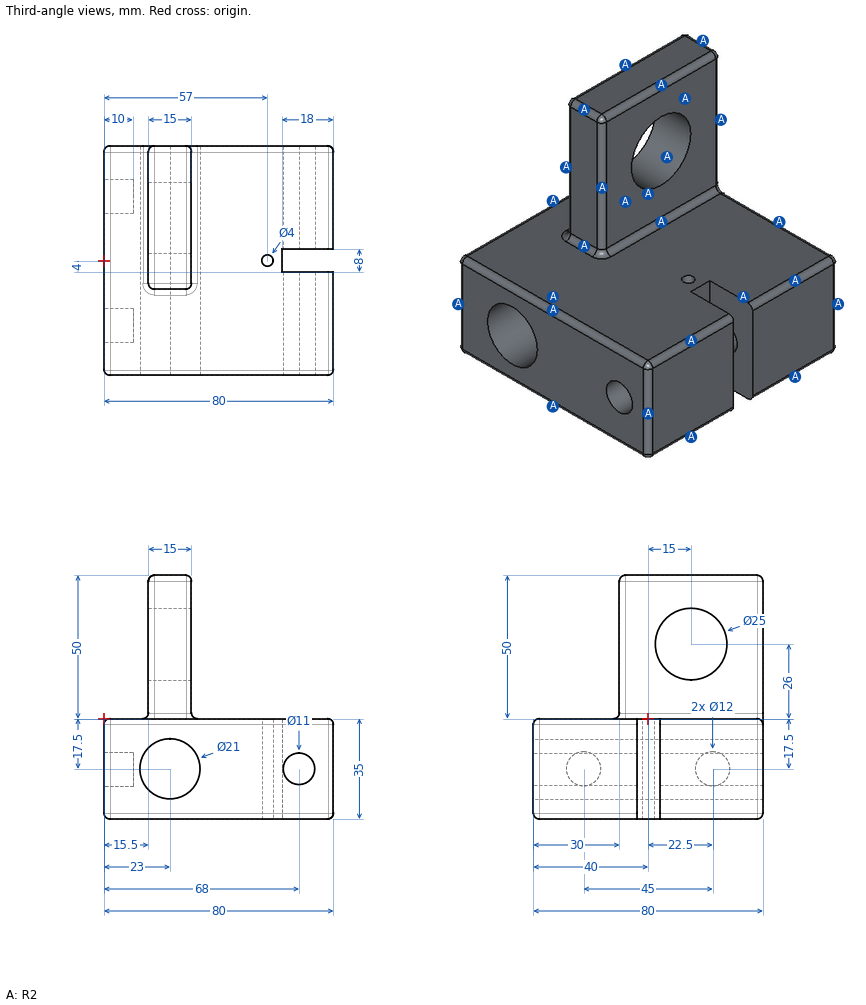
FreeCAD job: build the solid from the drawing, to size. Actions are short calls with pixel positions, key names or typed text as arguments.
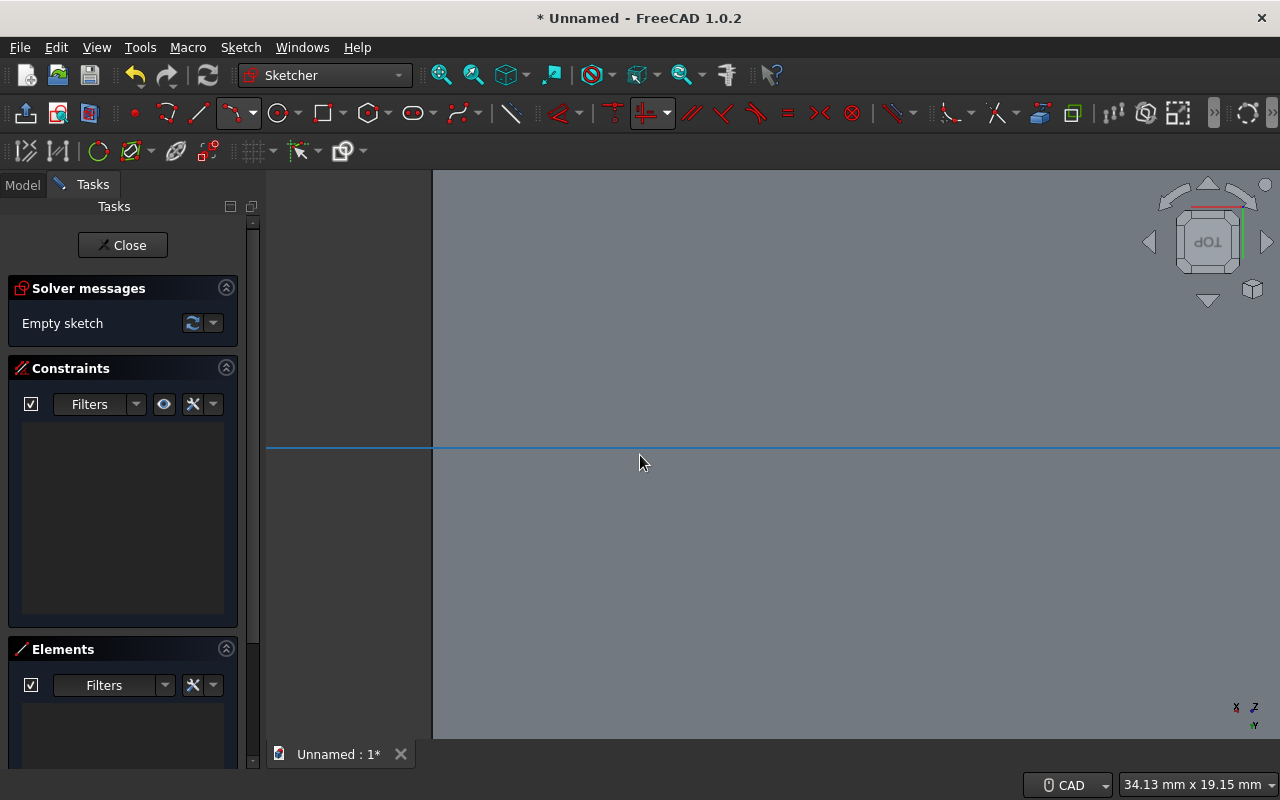
click(324, 114)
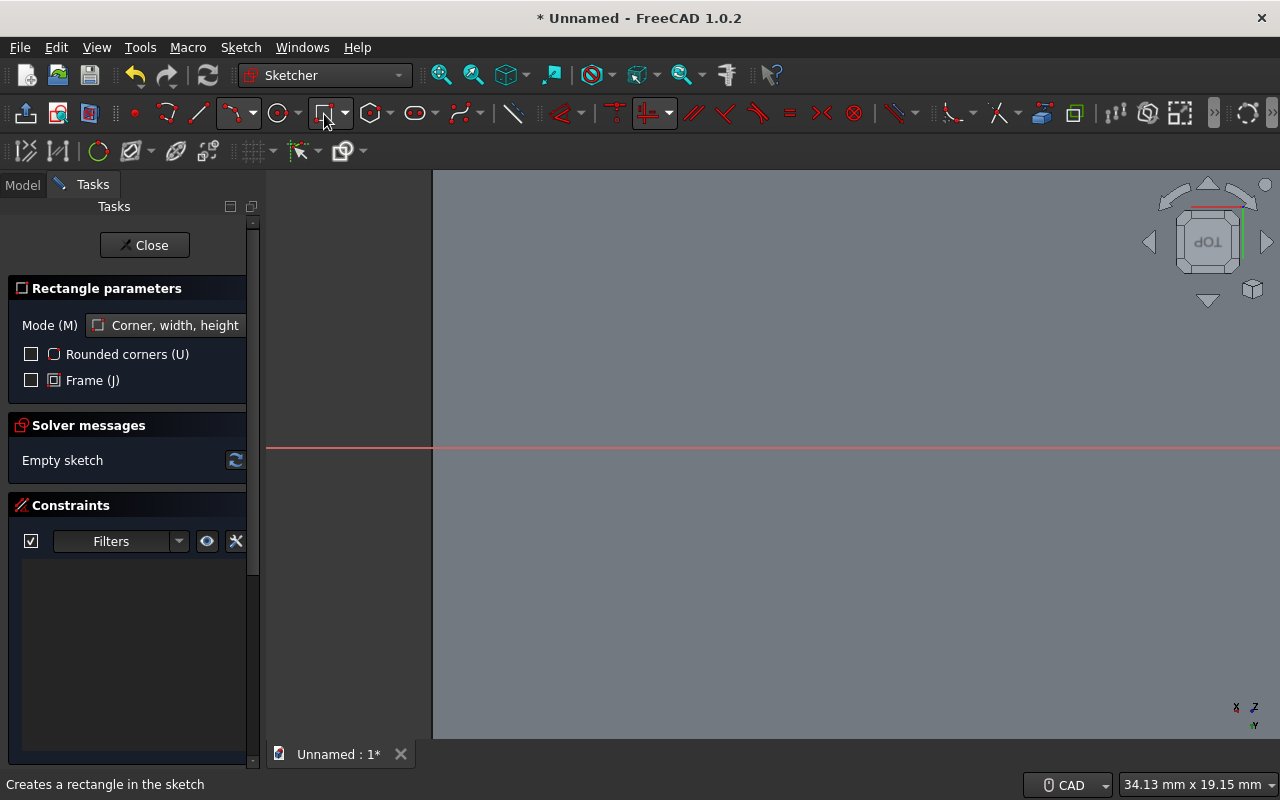
click(432, 329)
click(967, 567)
key(Escape)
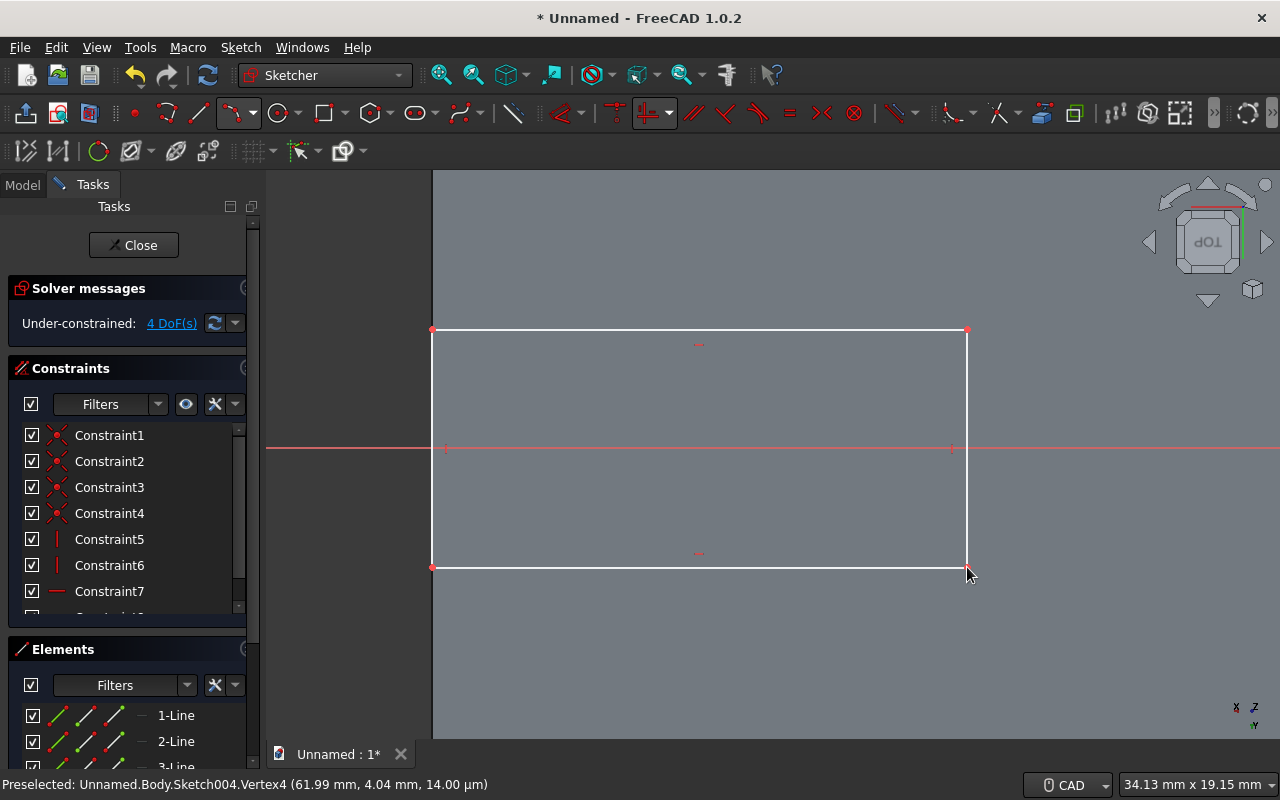
click(560, 114)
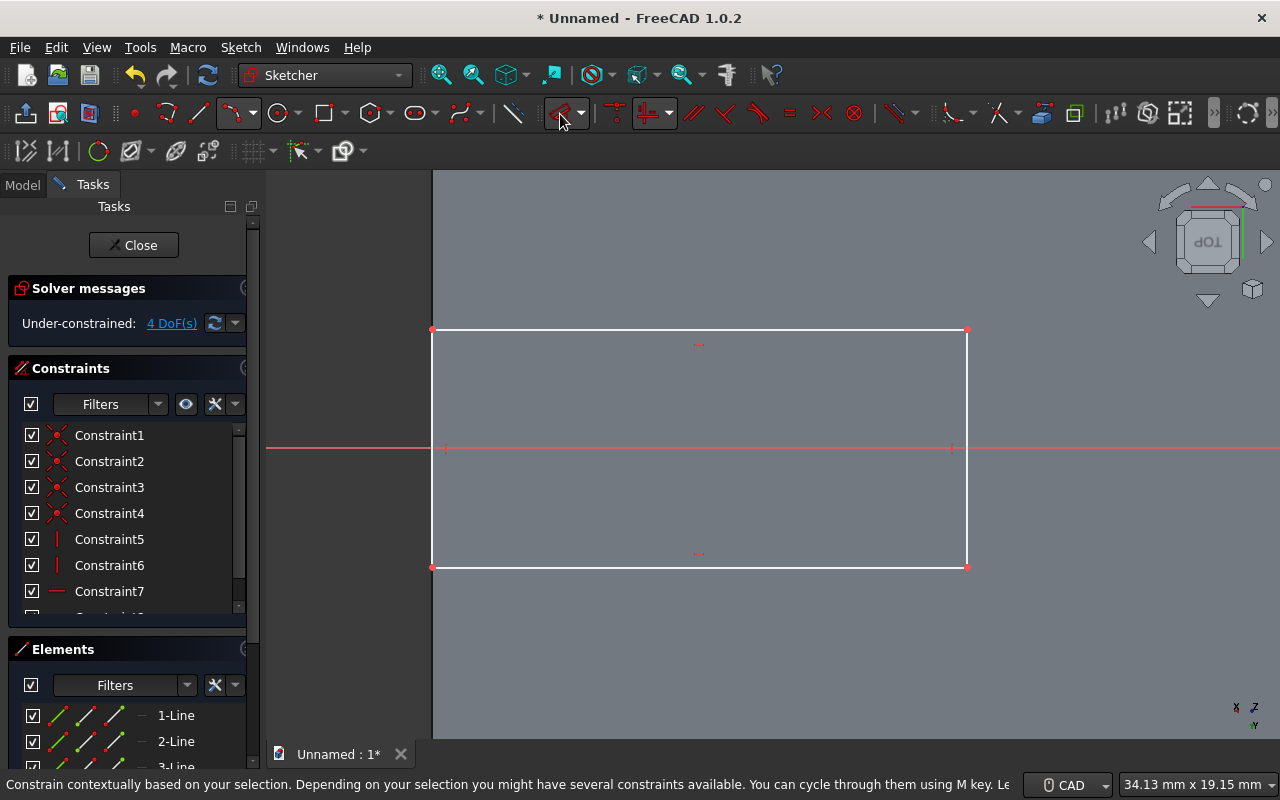
click(432, 401)
click(398, 394)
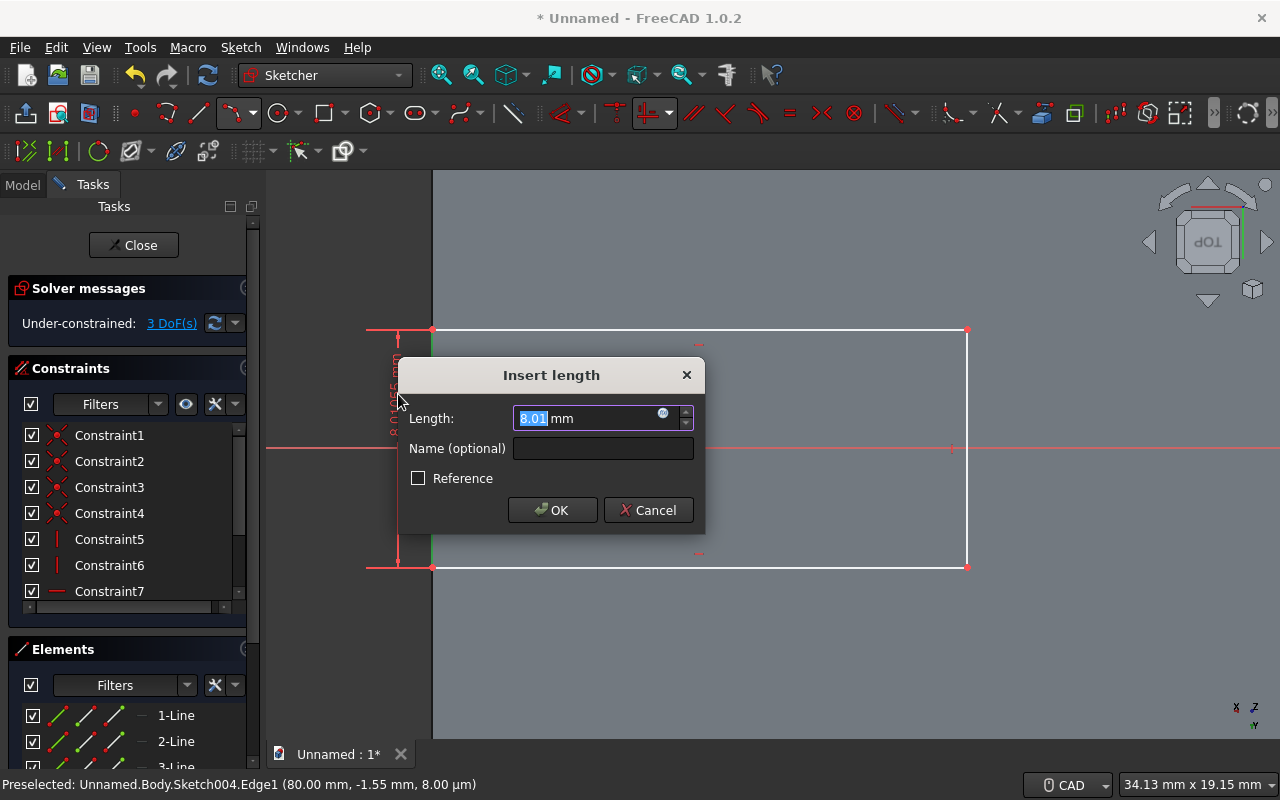
text(8)
key(Return)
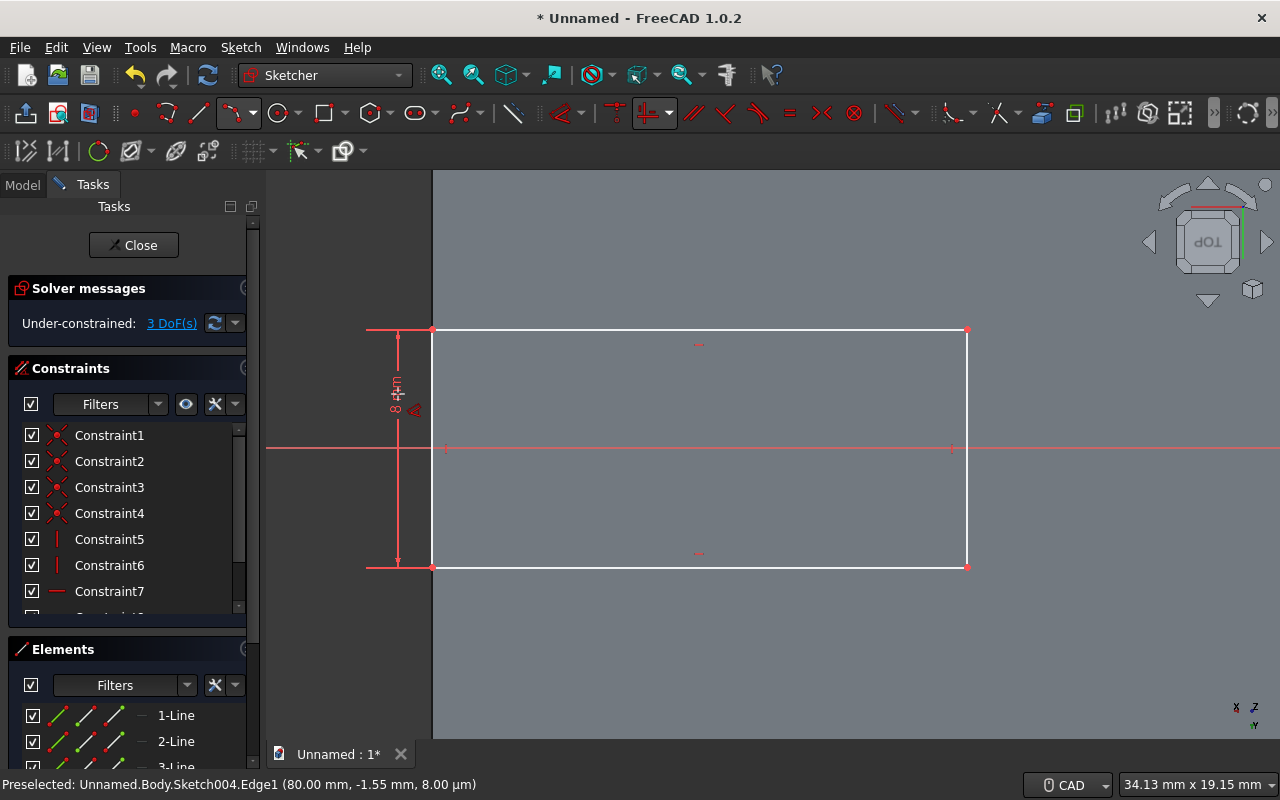
click(592, 568)
click(700, 602)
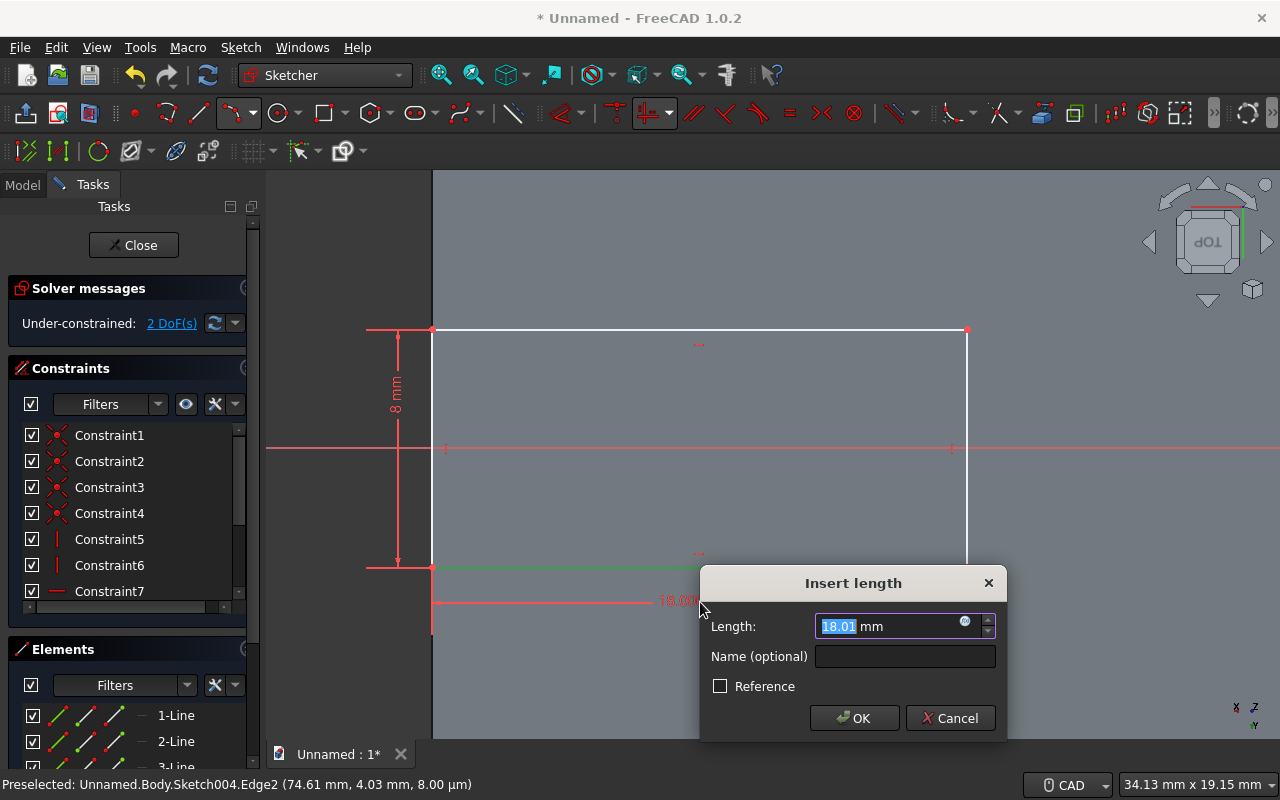
text(18)
key(Return)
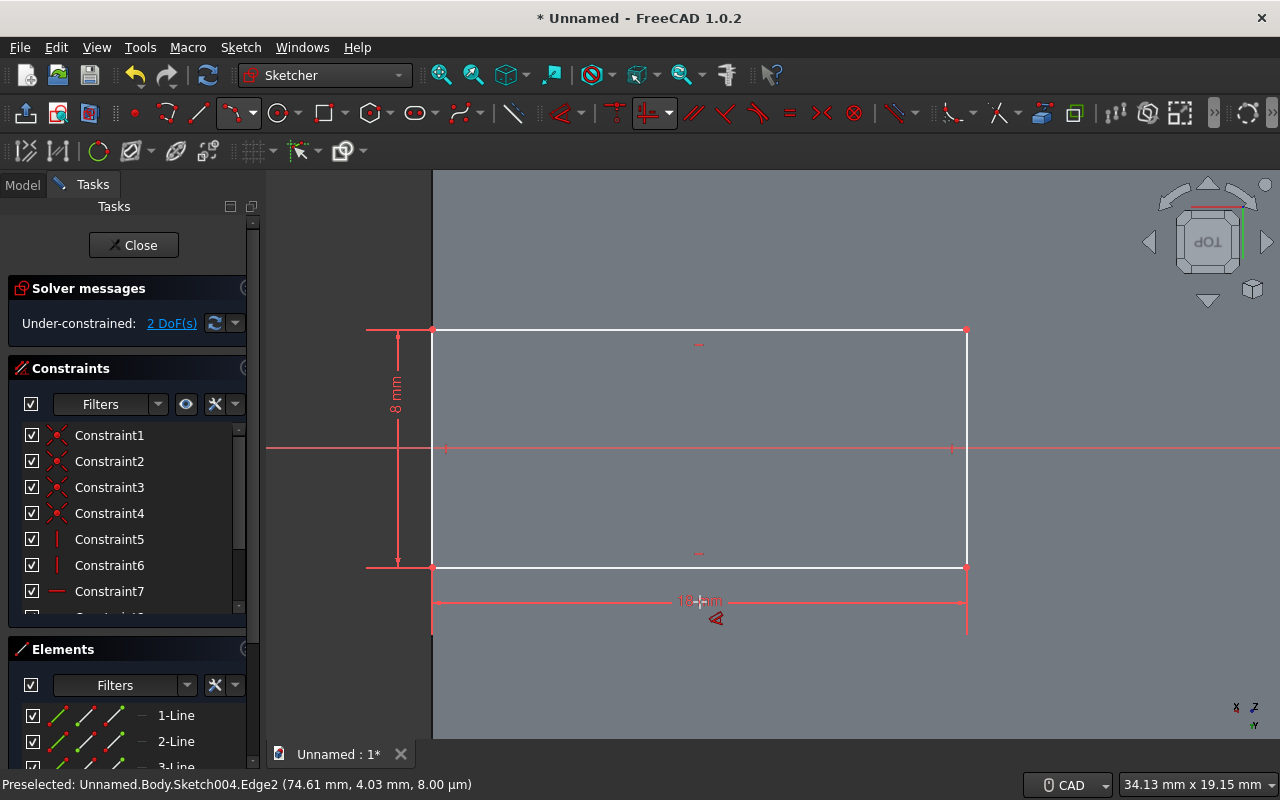
click(432, 330)
click(398, 362)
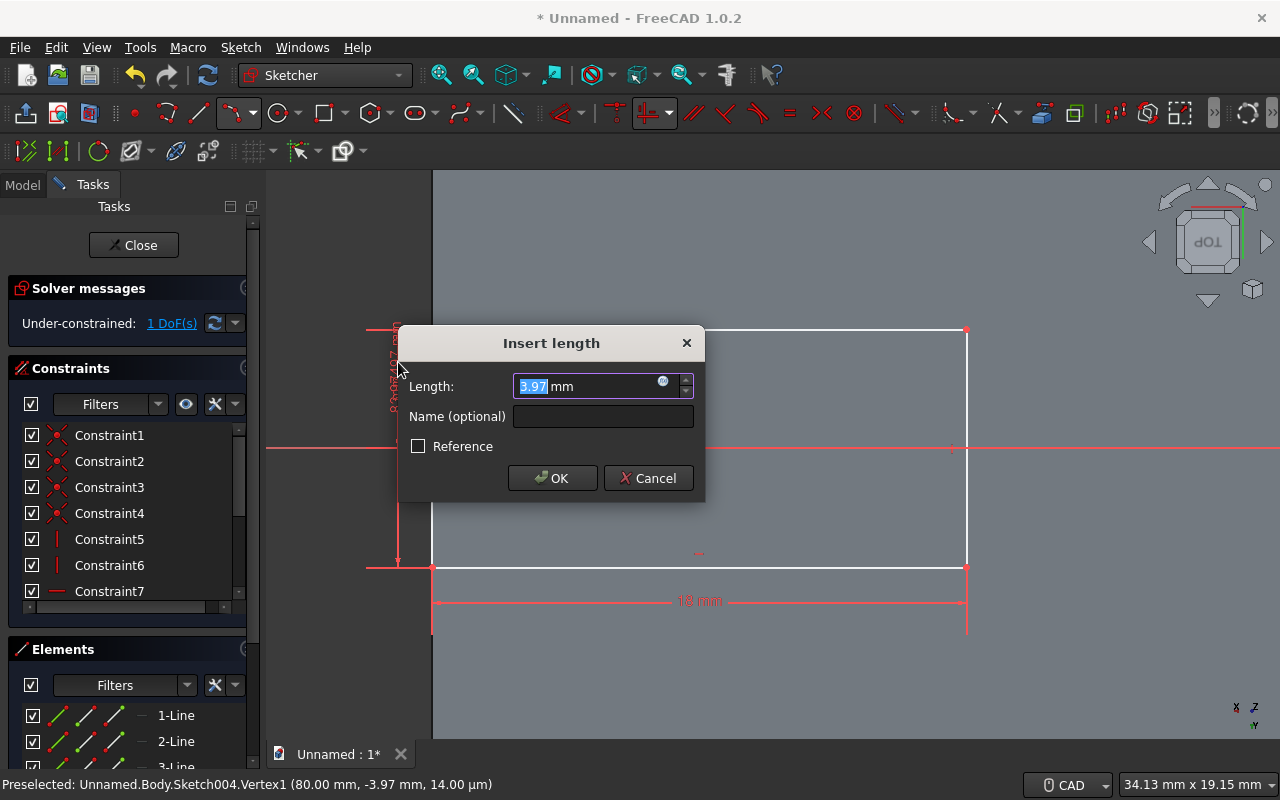
text(4)
key(Return)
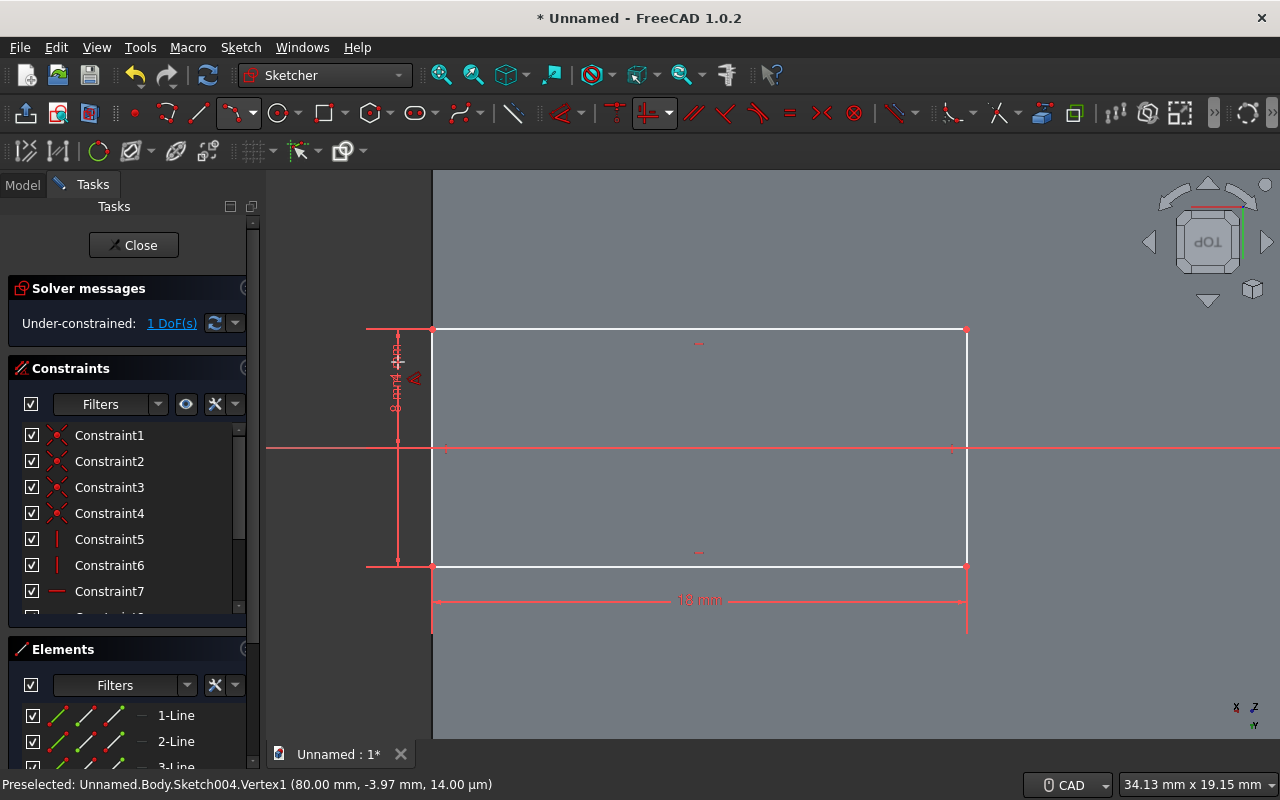
click(432, 329)
click(773, 295)